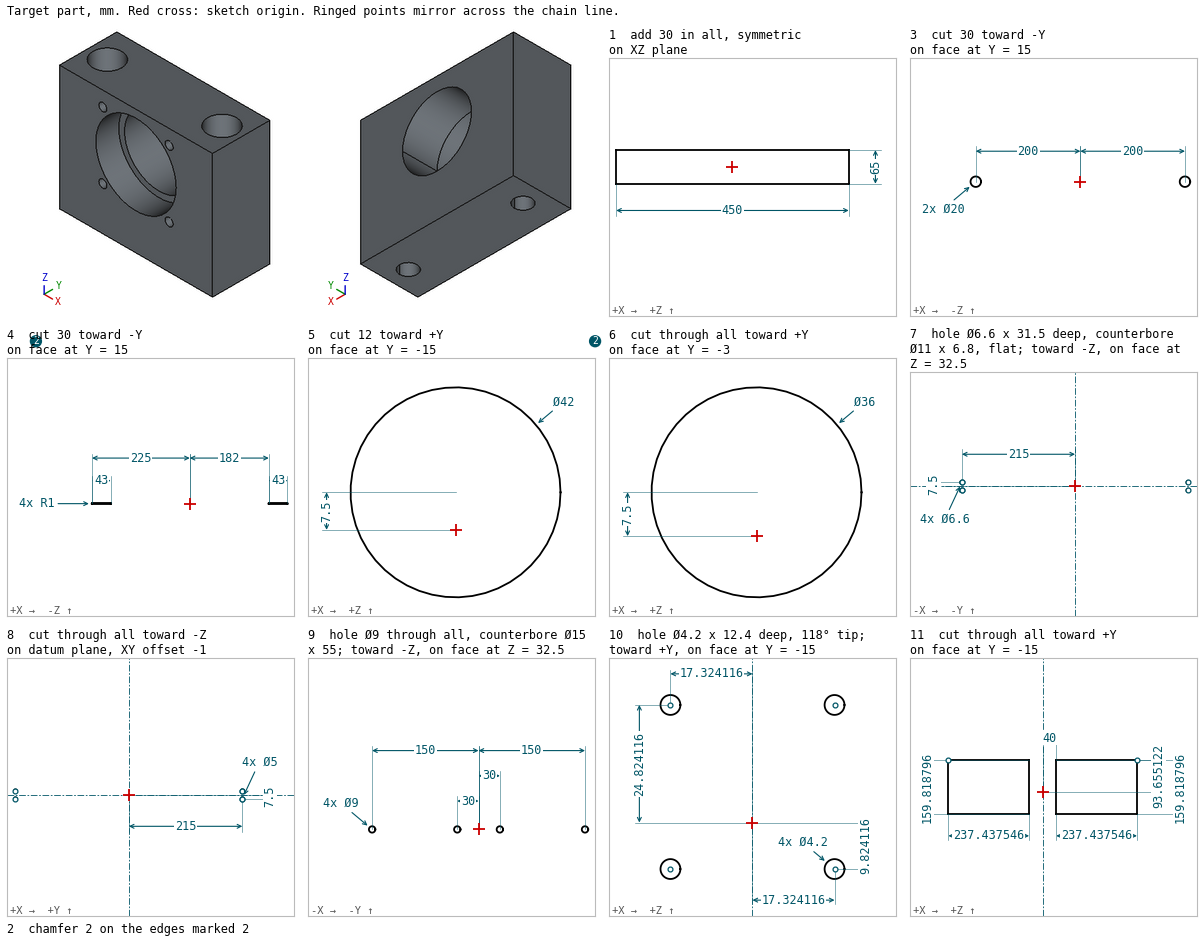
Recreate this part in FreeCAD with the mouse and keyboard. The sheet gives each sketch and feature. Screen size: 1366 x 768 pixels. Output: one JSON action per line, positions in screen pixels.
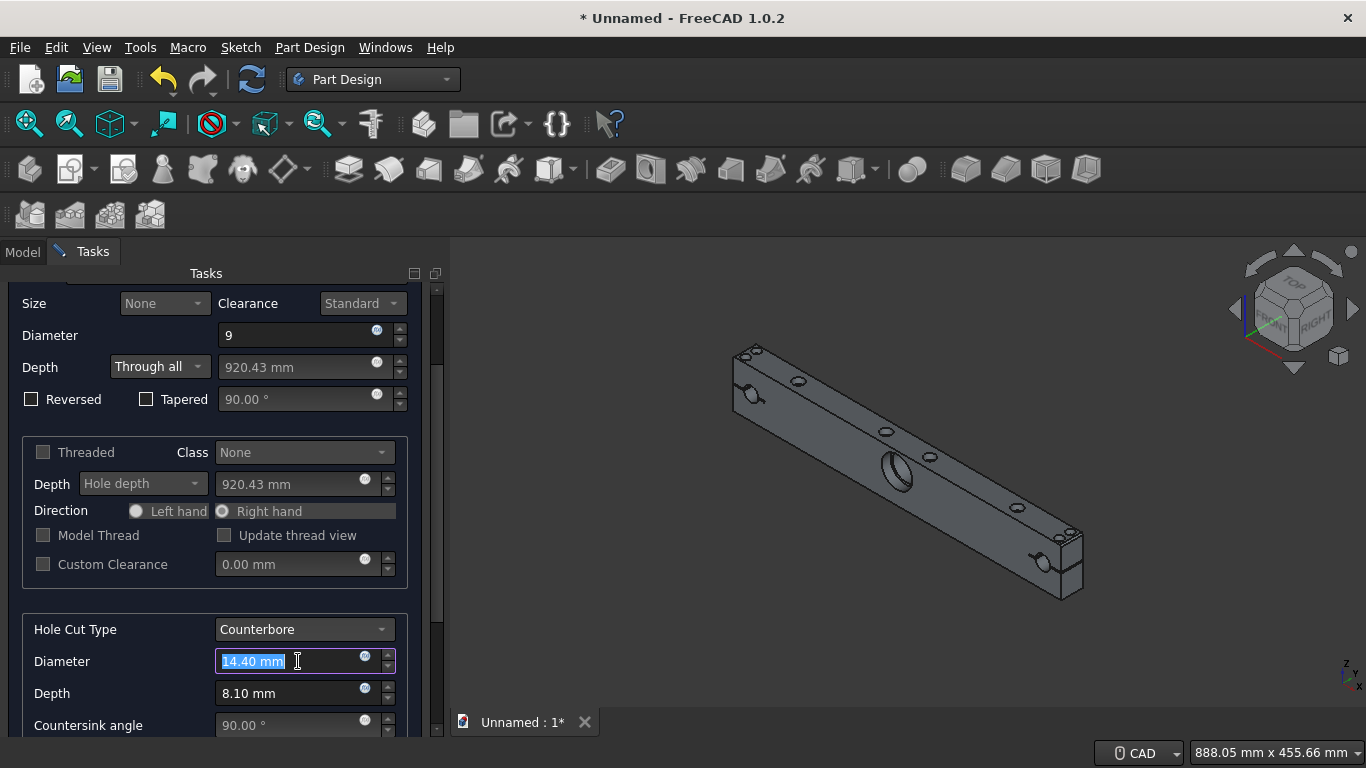
{"action": "type", "text": "15"}
{"action": "key", "text": "Tab"}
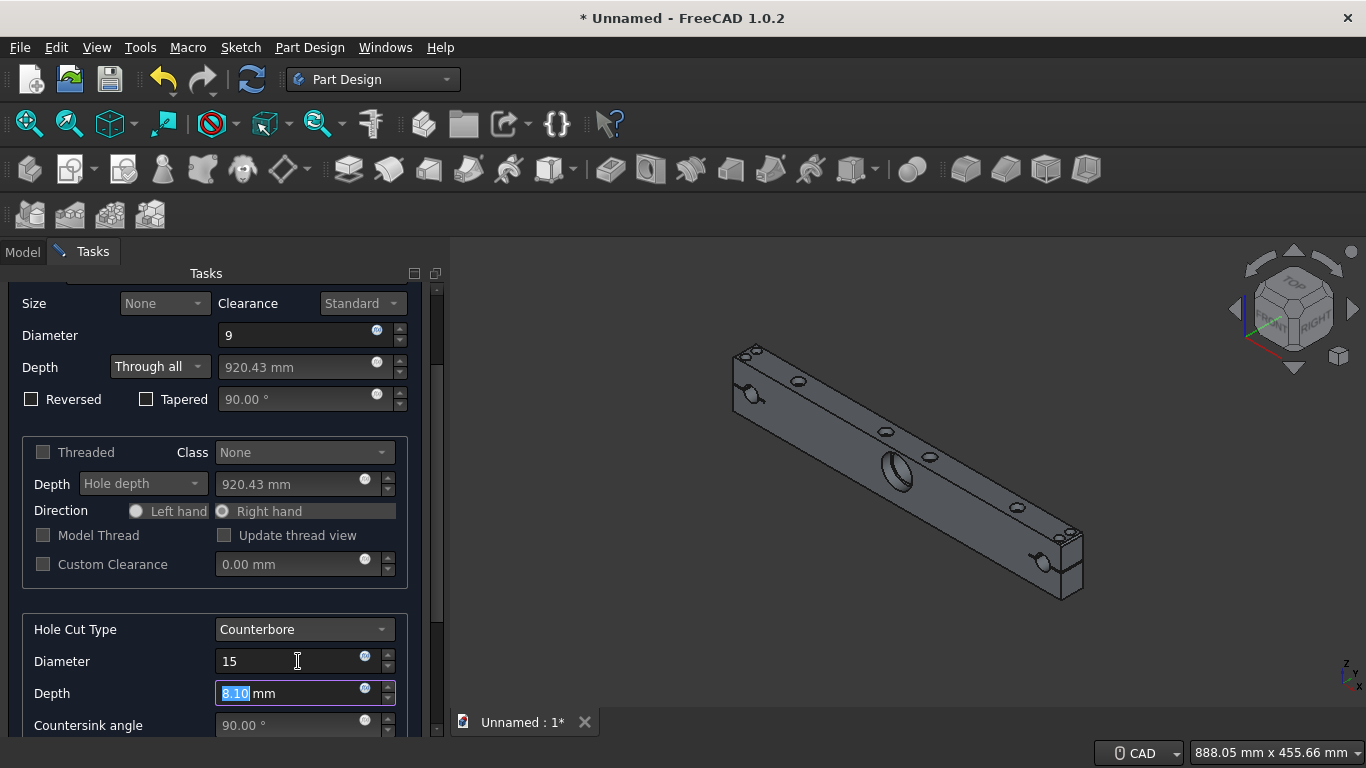
{"action": "type", "text": "55"}
{"action": "key", "text": "Tab"}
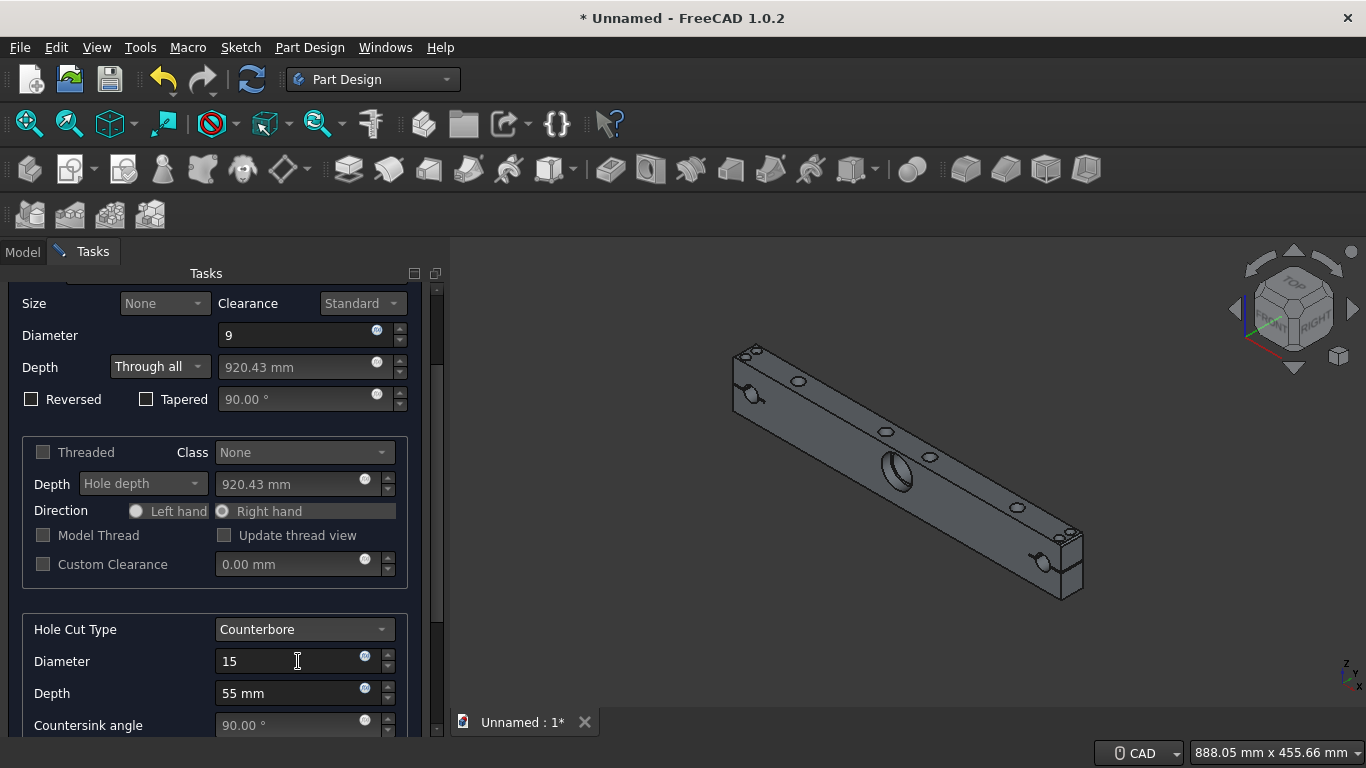
{"action": "scroll", "coordinate": [437, 510], "scroll_direction": "up", "scroll_amount": 3}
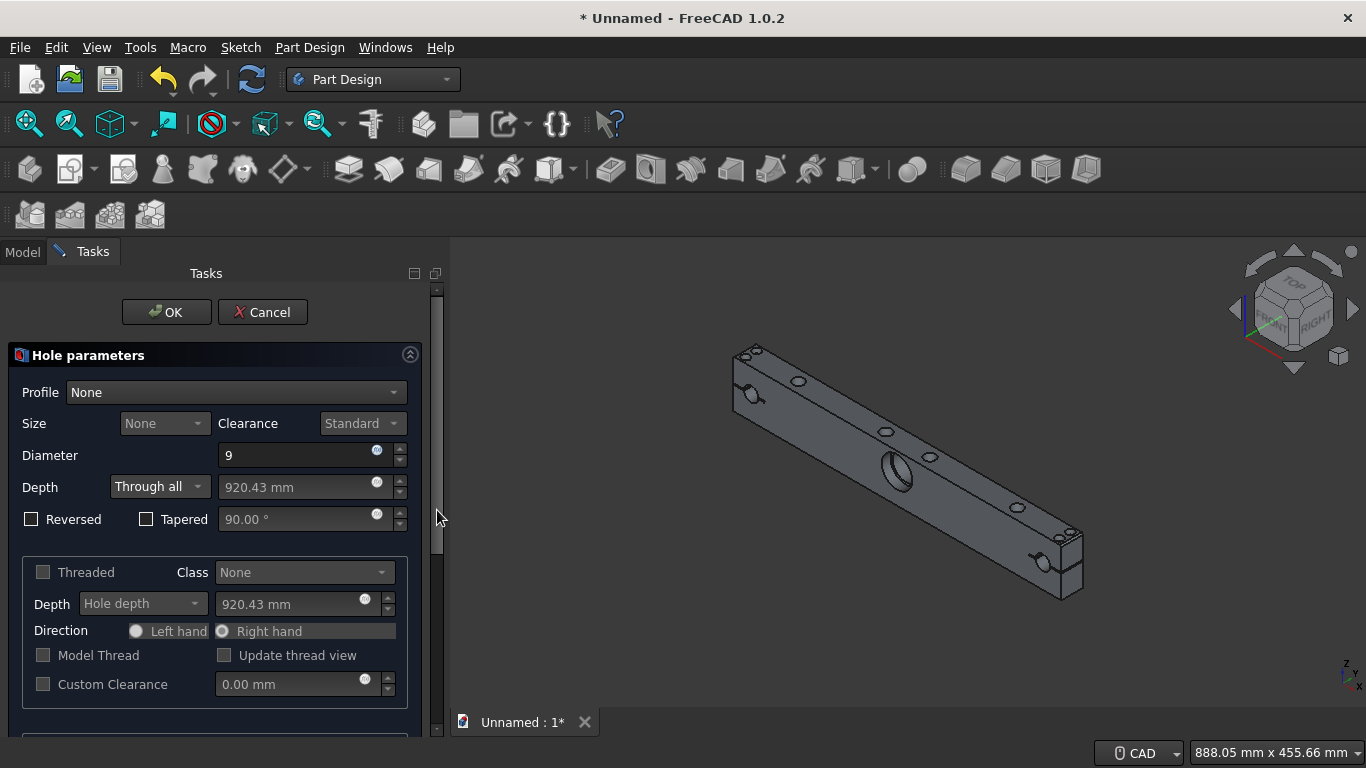
{"action": "left_click", "coordinate": [167, 312]}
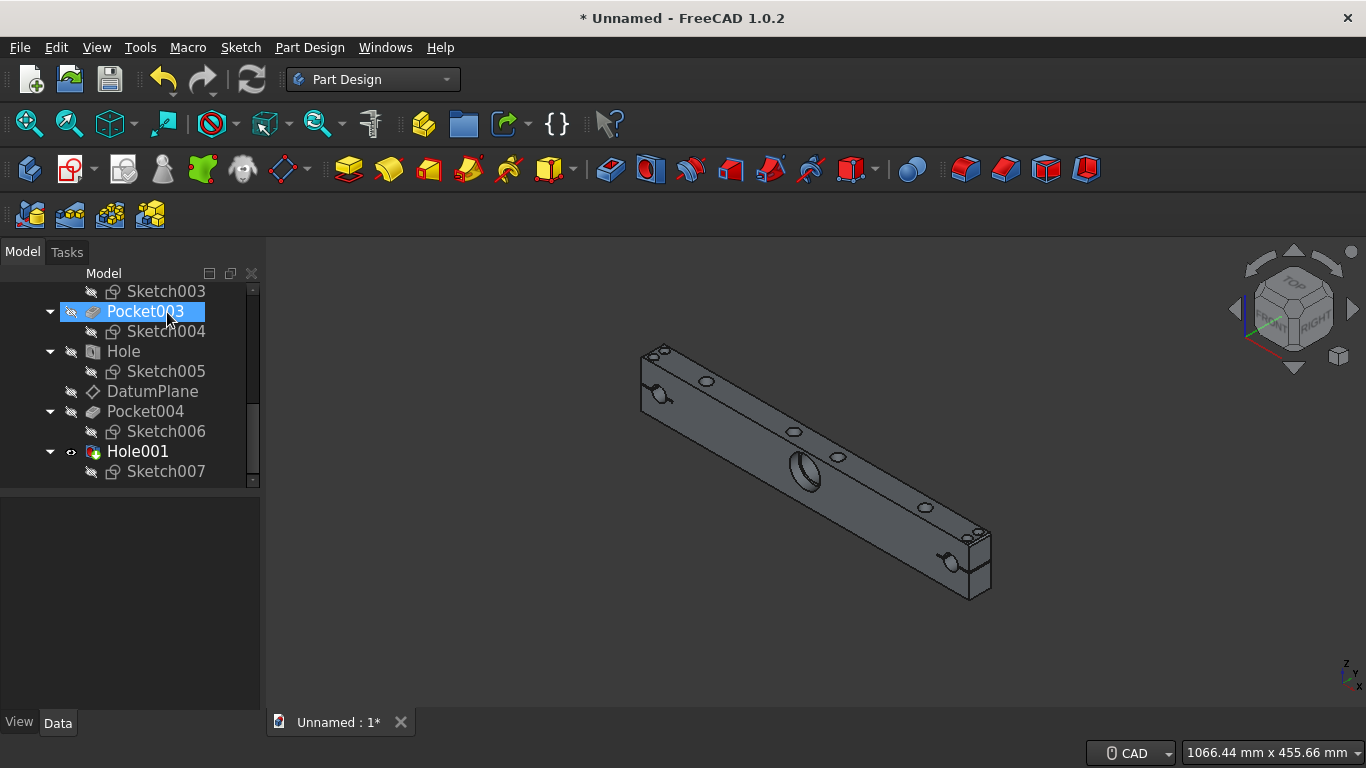
{"action": "left_click", "coordinate": [899, 531]}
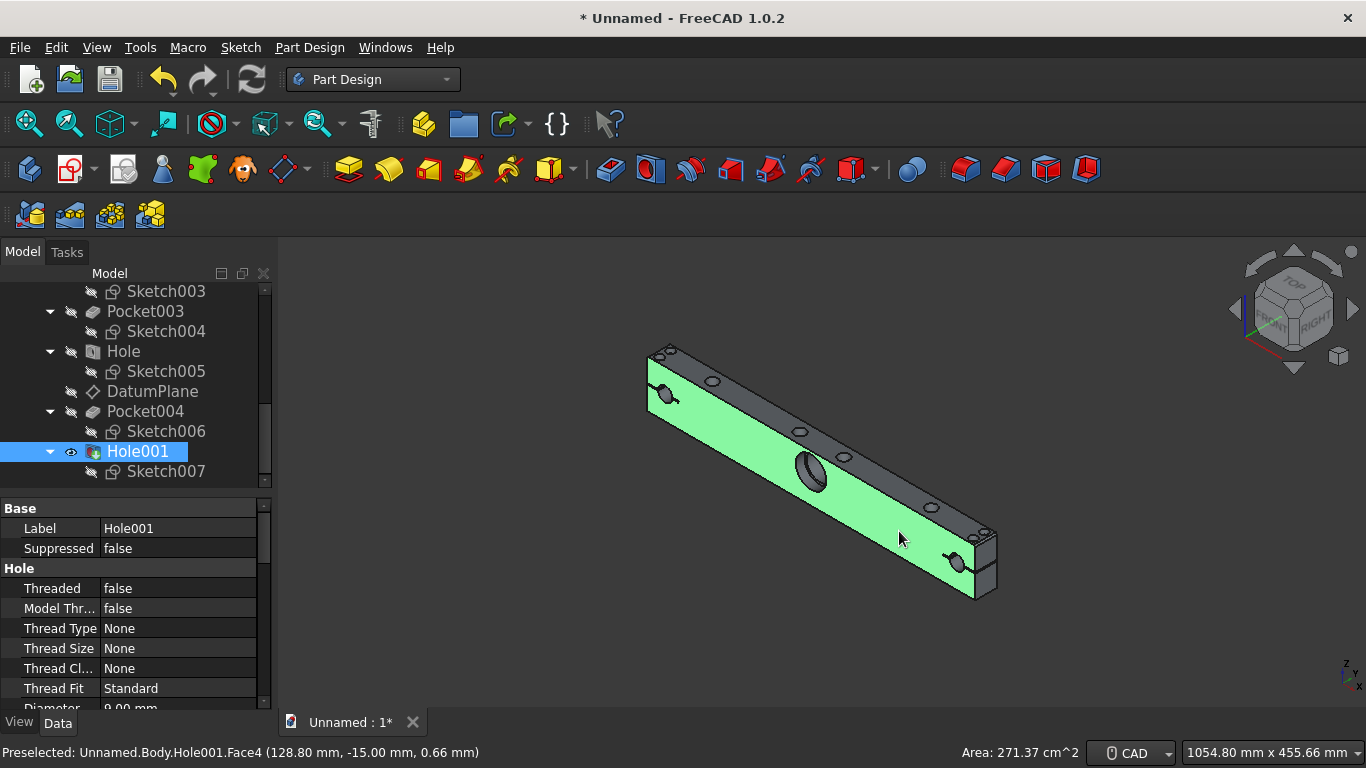
{"action": "left_click", "coordinate": [70, 170]}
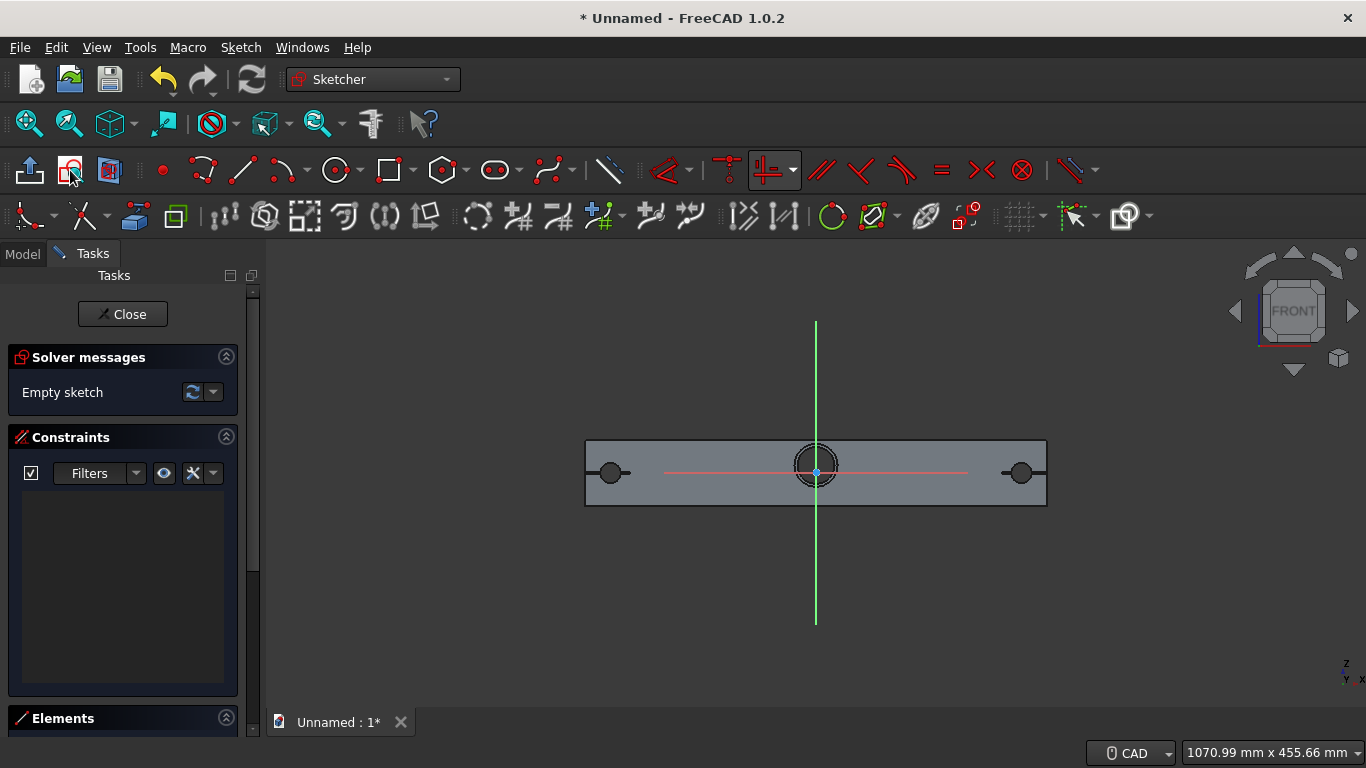
{"action": "scroll", "coordinate": [827, 464], "scroll_direction": "up", "scroll_amount": 10}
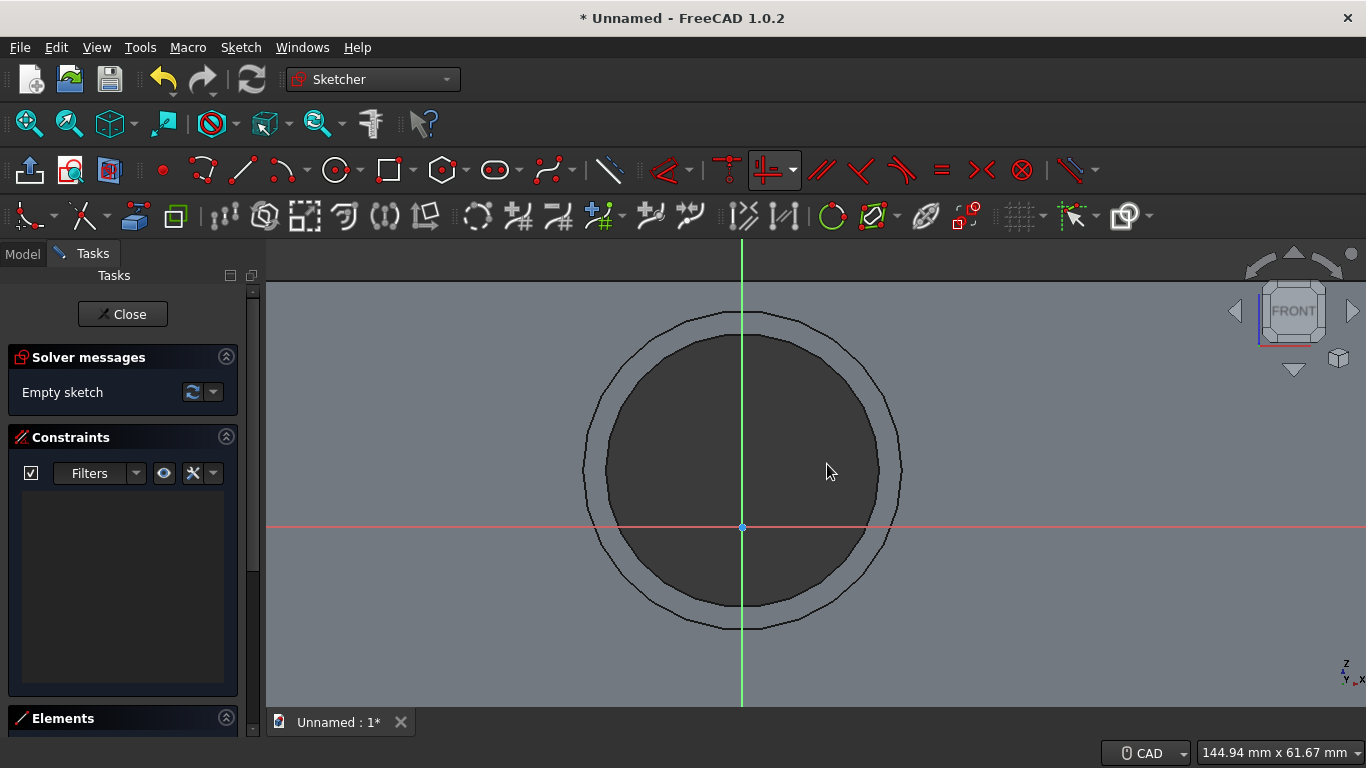
{"action": "key", "text": "g c"}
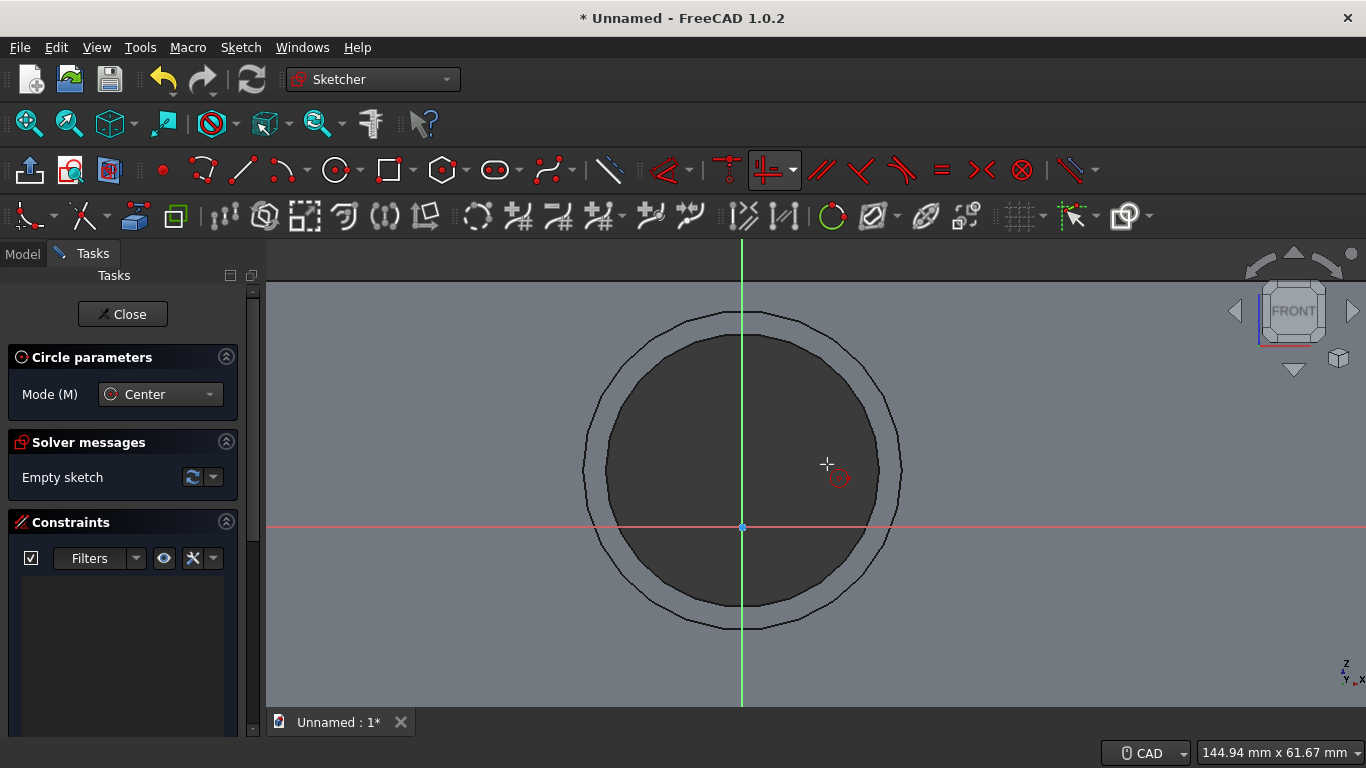
{"action": "scroll", "coordinate": [874, 602], "scroll_direction": "up", "scroll_amount": 2}